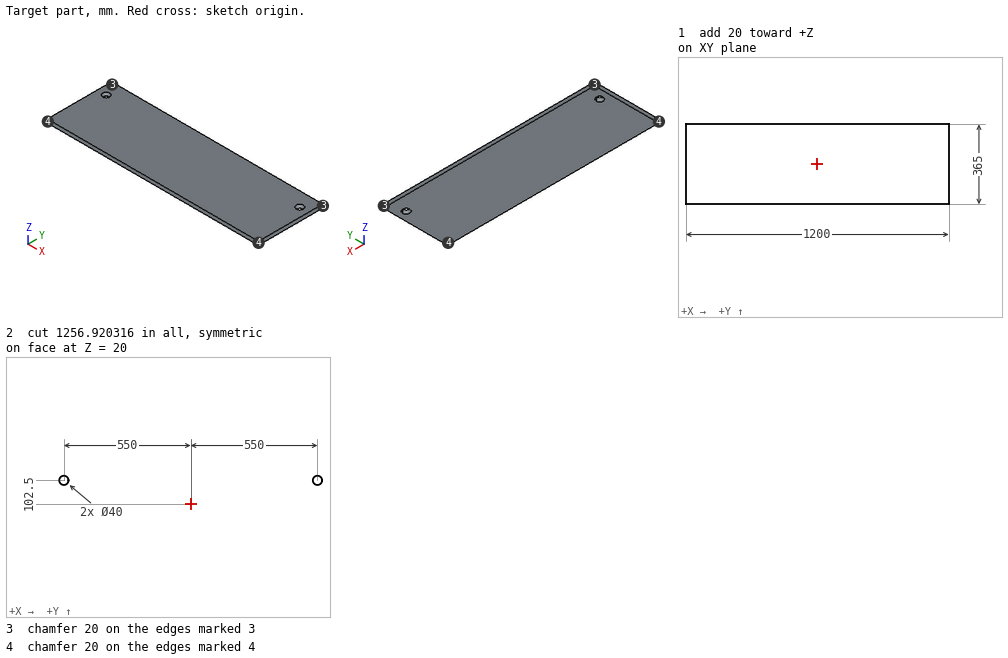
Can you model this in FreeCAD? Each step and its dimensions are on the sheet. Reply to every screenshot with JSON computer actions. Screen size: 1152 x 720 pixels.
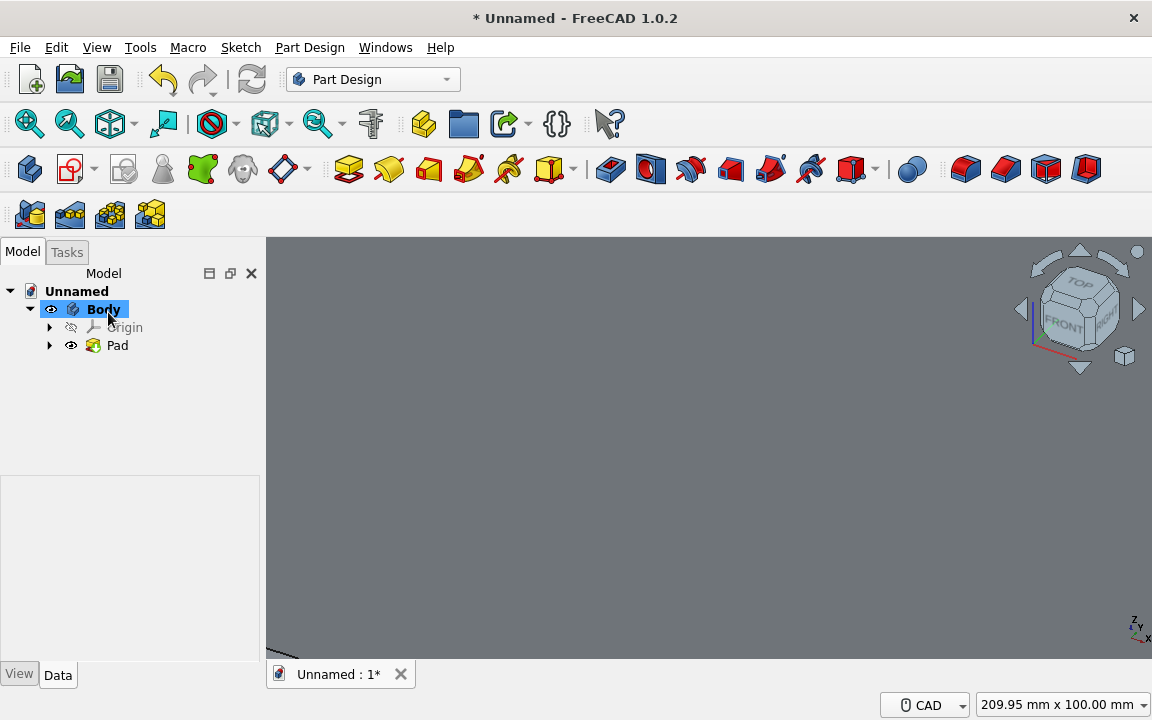
{"action": "key", "text": "v f"}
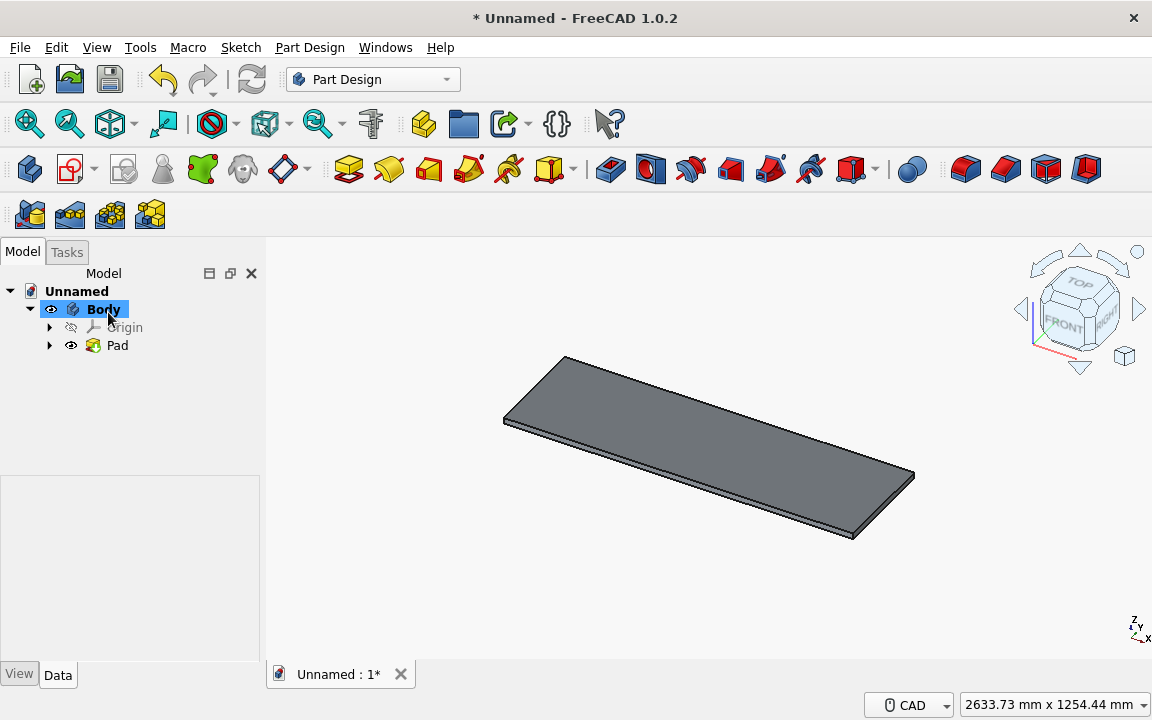
{"action": "left_click", "coordinate": [809, 477]}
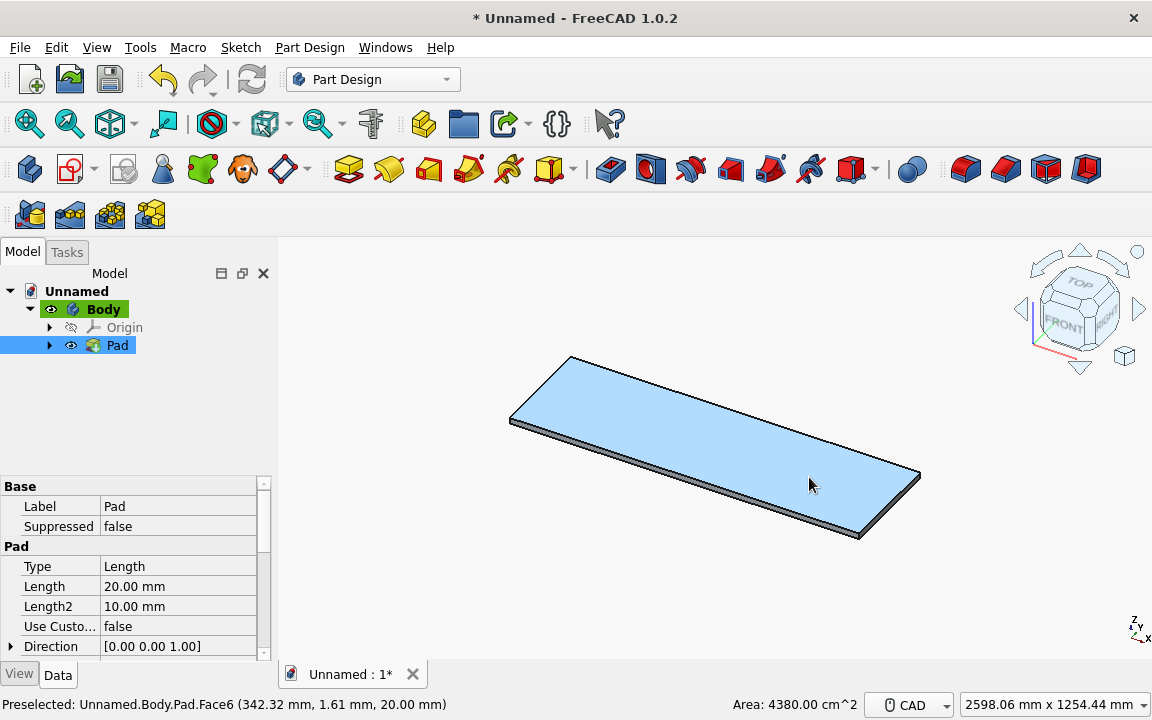
{"action": "left_click", "coordinate": [70, 170]}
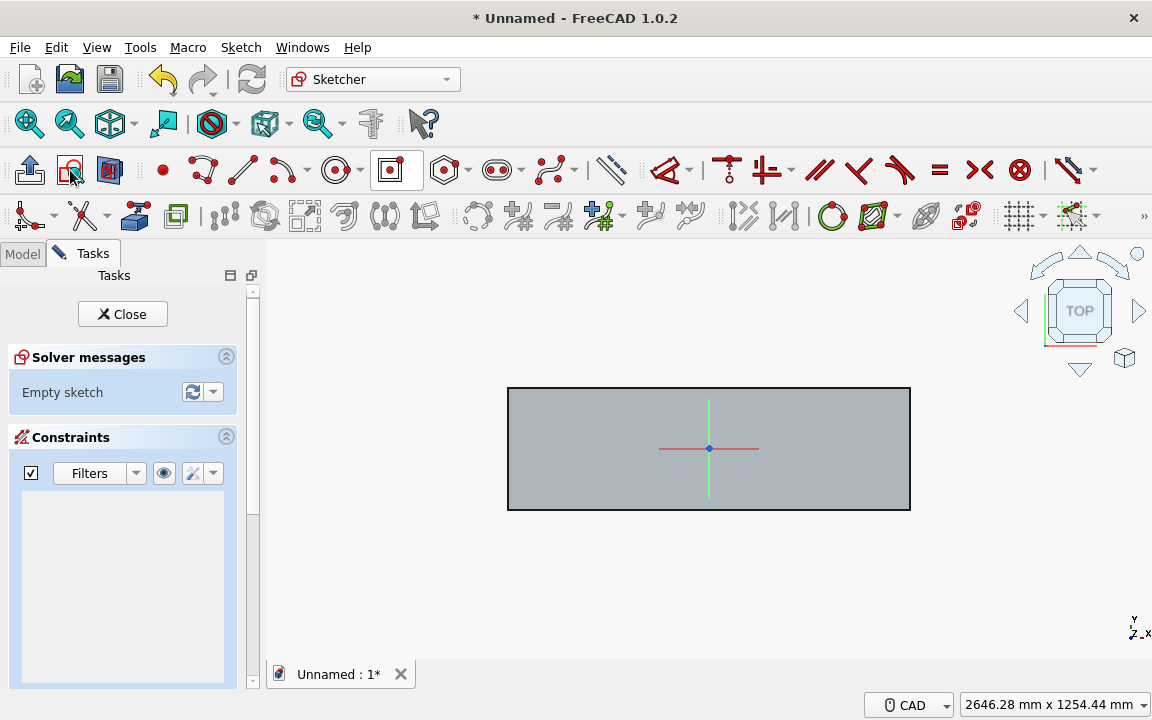
{"action": "key", "text": "g c"}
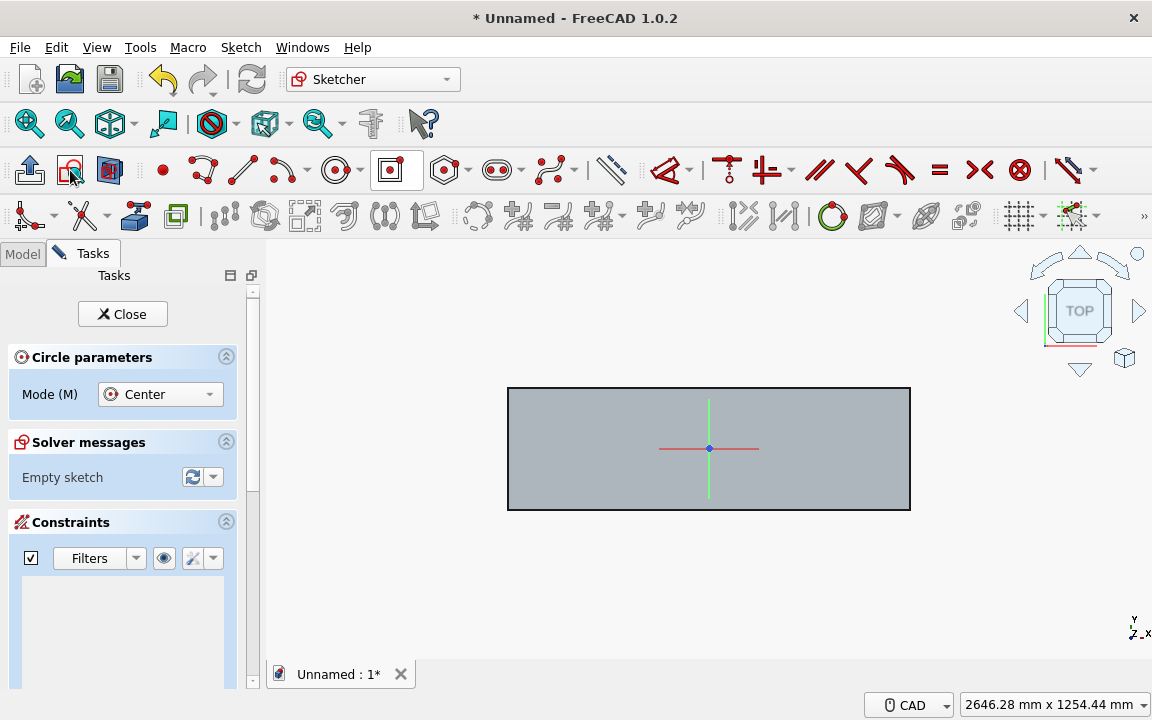
{"action": "scroll", "coordinate": [525, 415], "scroll_direction": "up", "scroll_amount": 7}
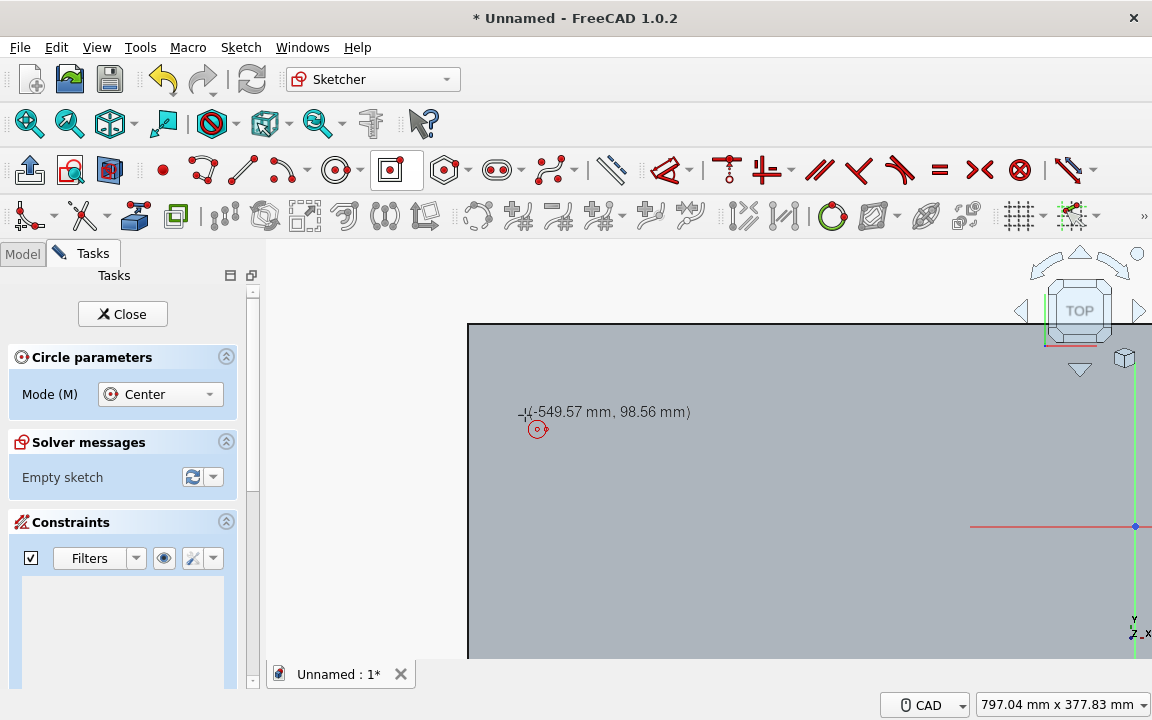
{"action": "scroll", "coordinate": [369, 441], "scroll_direction": "down", "scroll_amount": 6}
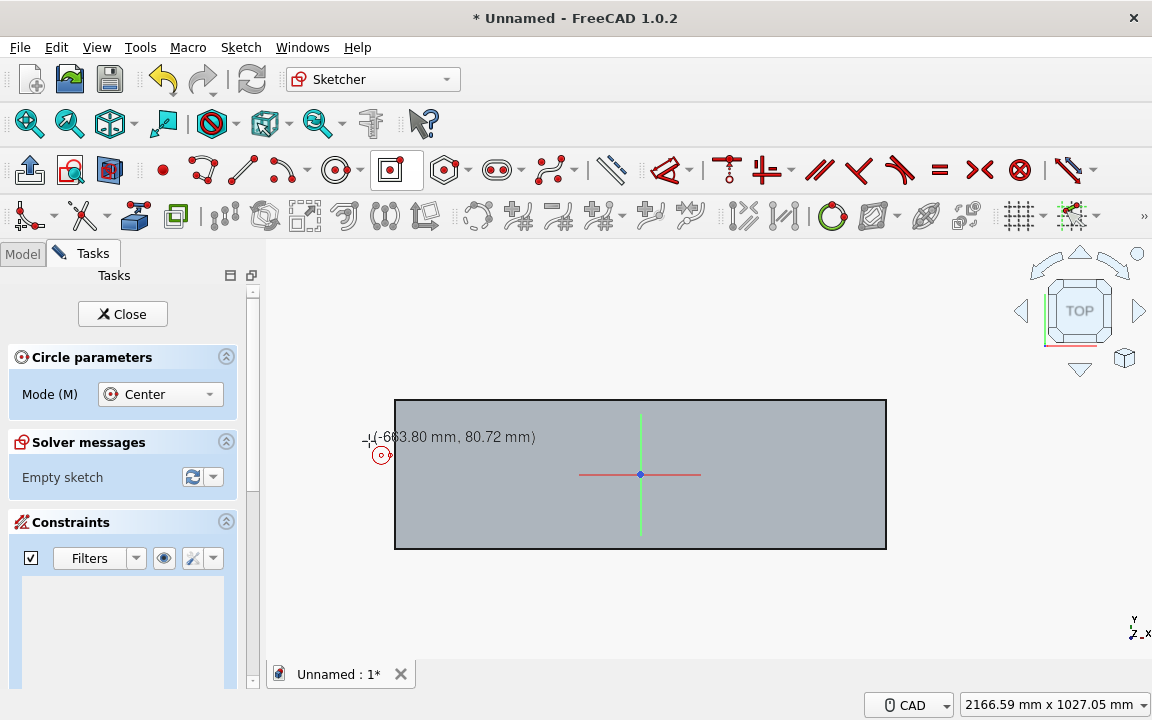
{"action": "left_click", "coordinate": [416, 433]}
{"action": "mouse_move", "coordinate": [421, 427]}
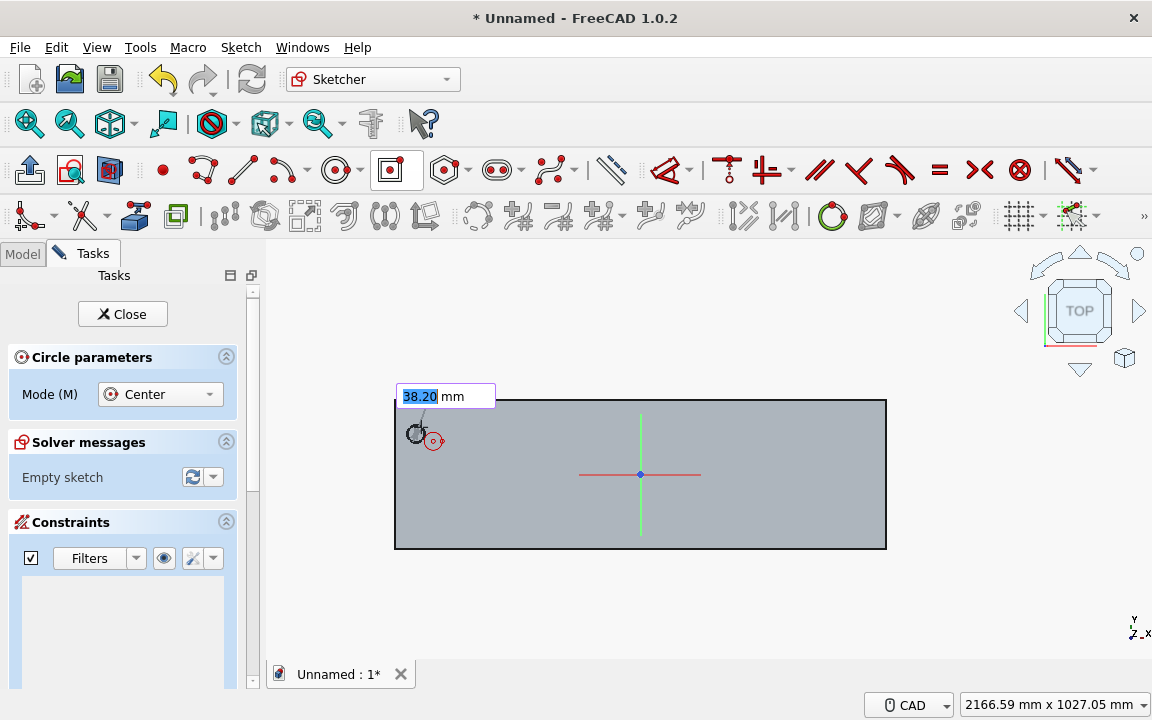
{"action": "type", "text": "40"}
{"action": "key", "text": "Return"}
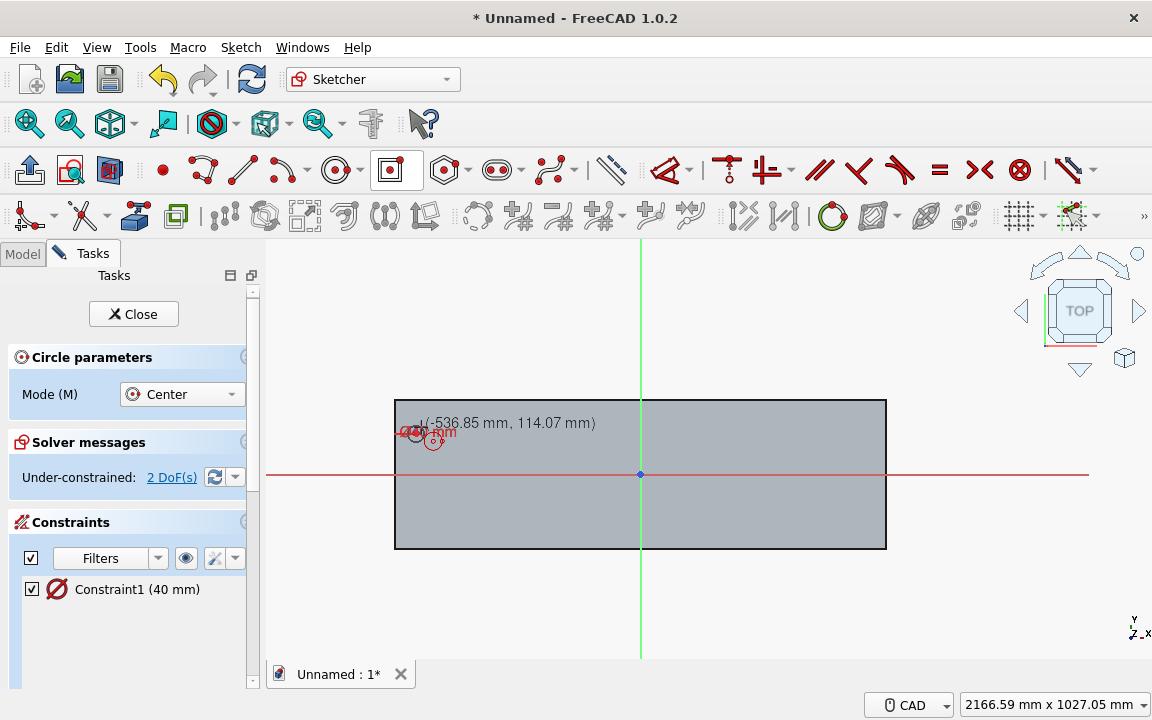
{"action": "scroll", "coordinate": [865, 433], "scroll_direction": "up", "scroll_amount": 6}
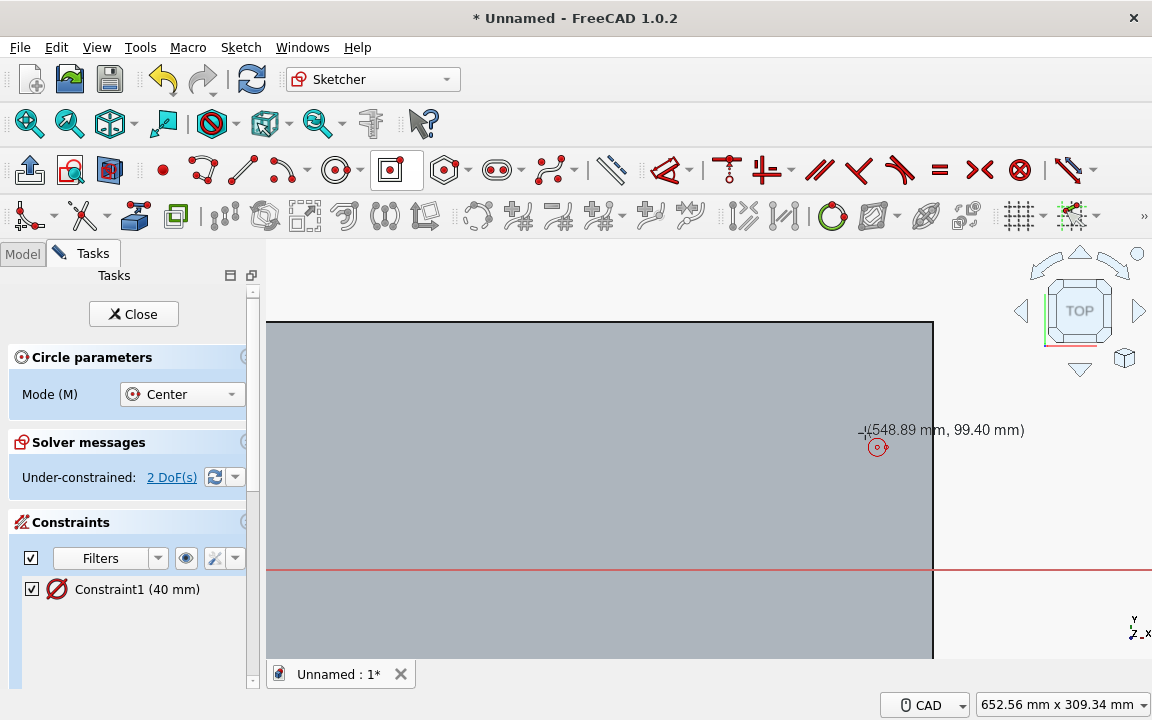
{"action": "scroll", "coordinate": [866, 433], "scroll_direction": "down", "scroll_amount": 6}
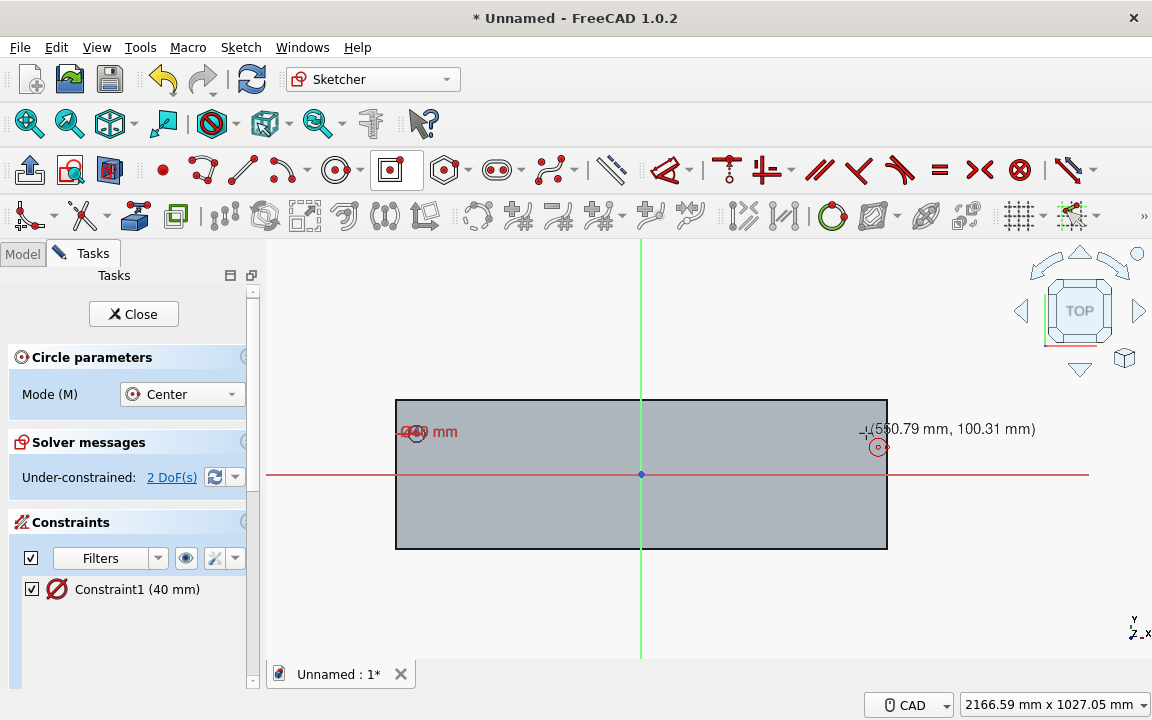
{"action": "left_click", "coordinate": [866, 433]}
{"action": "mouse_move", "coordinate": [872, 427]}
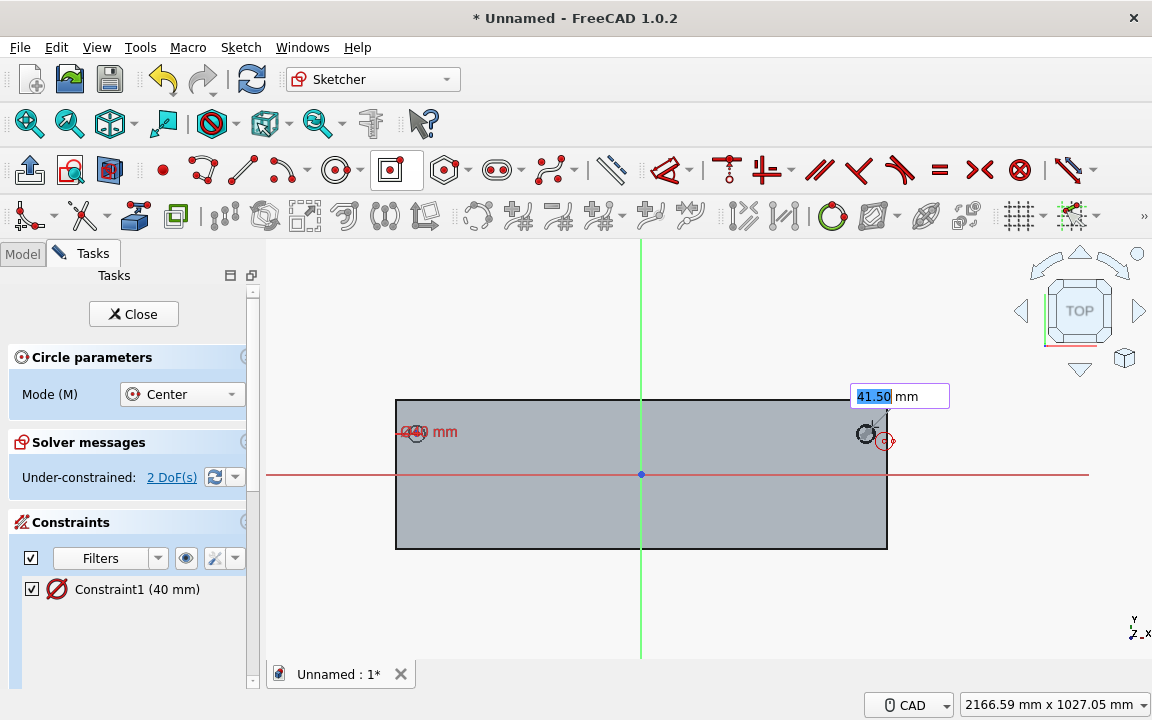
{"action": "type", "text": "40"}
{"action": "key", "text": "Return"}
{"action": "key", "text": "Escape"}